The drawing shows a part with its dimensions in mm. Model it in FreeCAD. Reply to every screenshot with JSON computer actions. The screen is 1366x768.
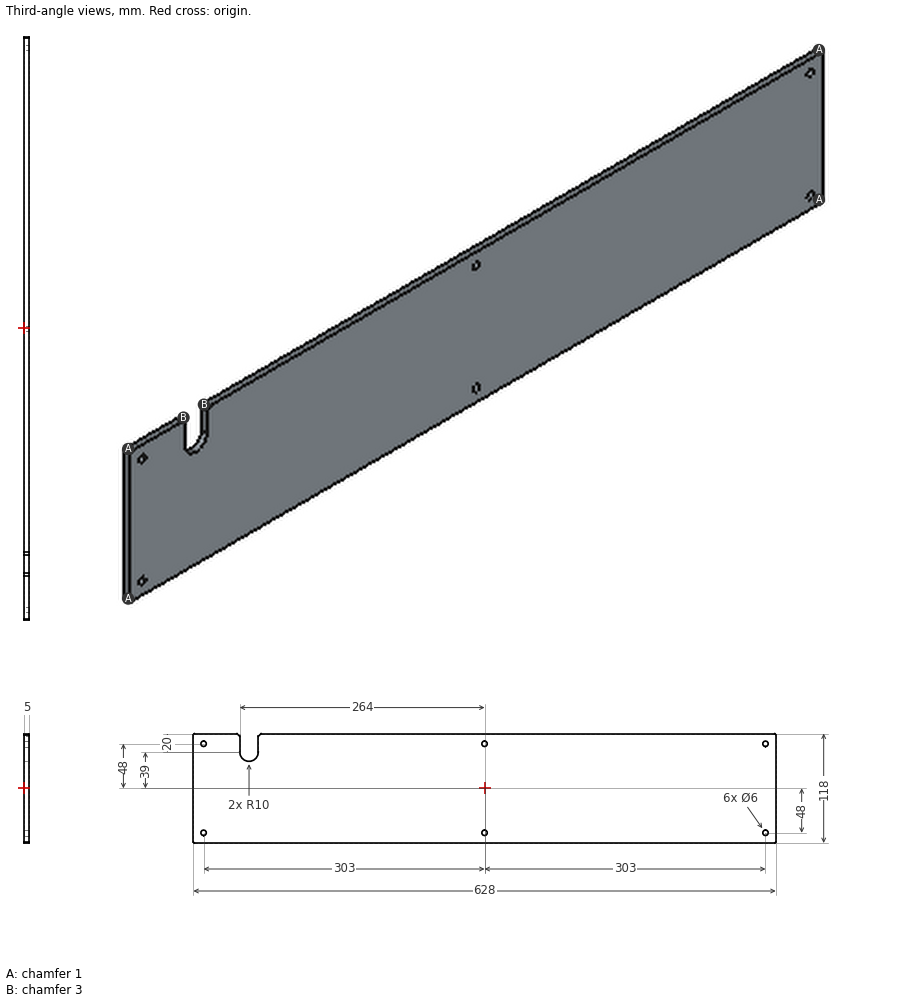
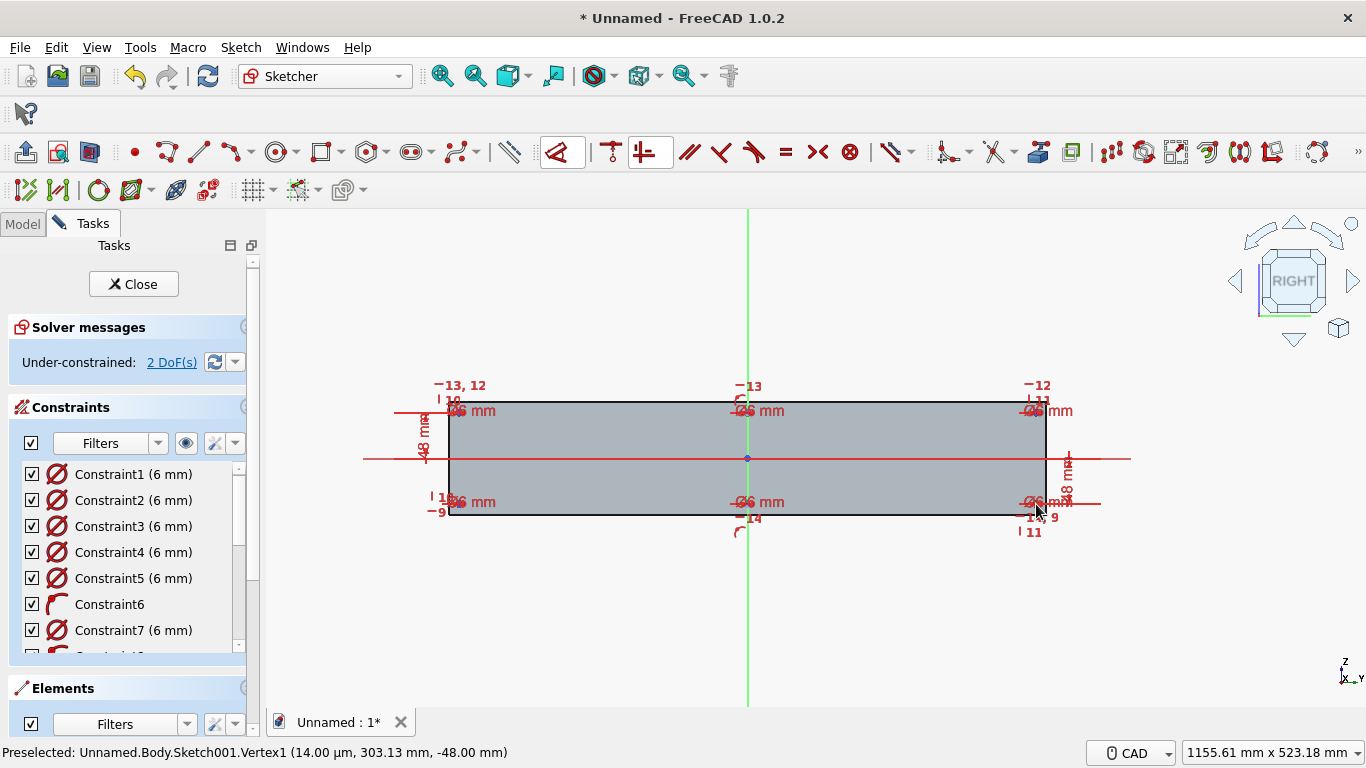
{"action": "left_click", "coordinate": [580, 152]}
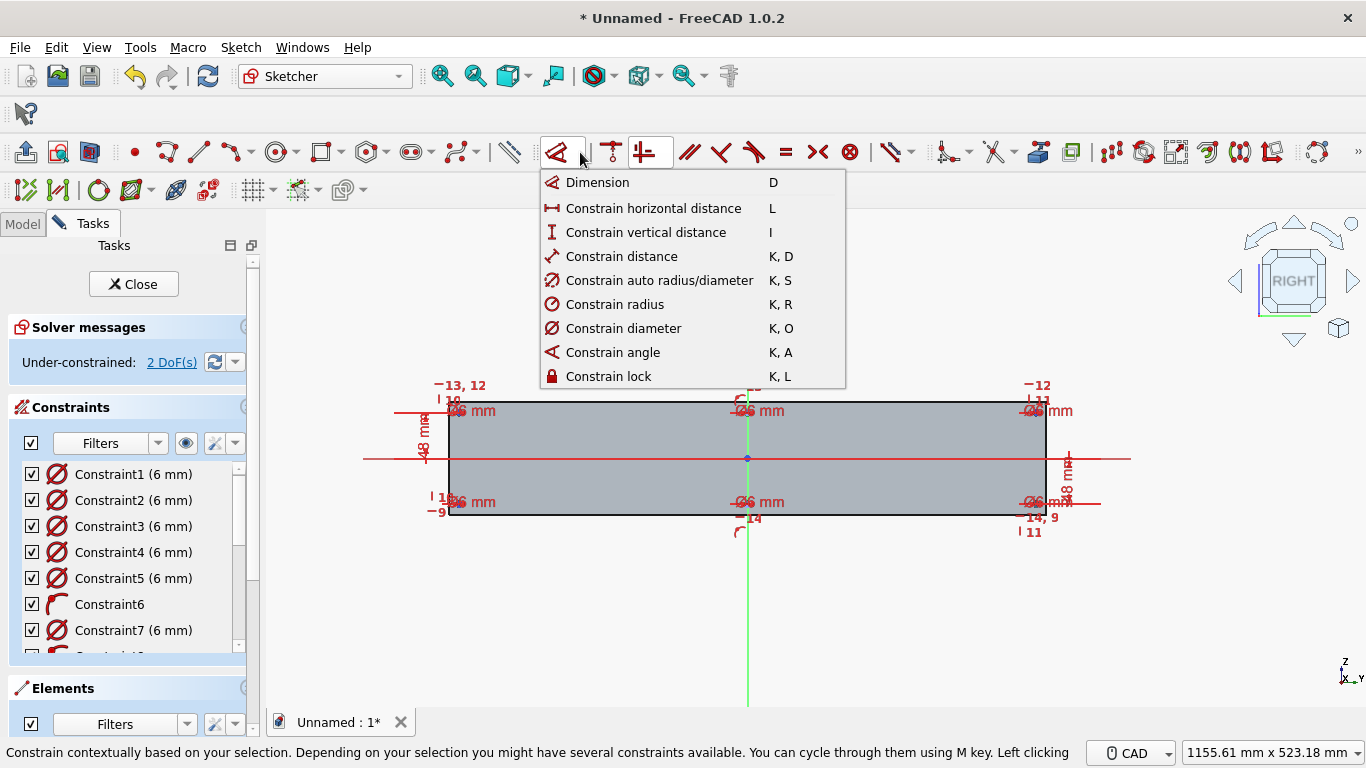
{"action": "left_click", "coordinate": [693, 208]}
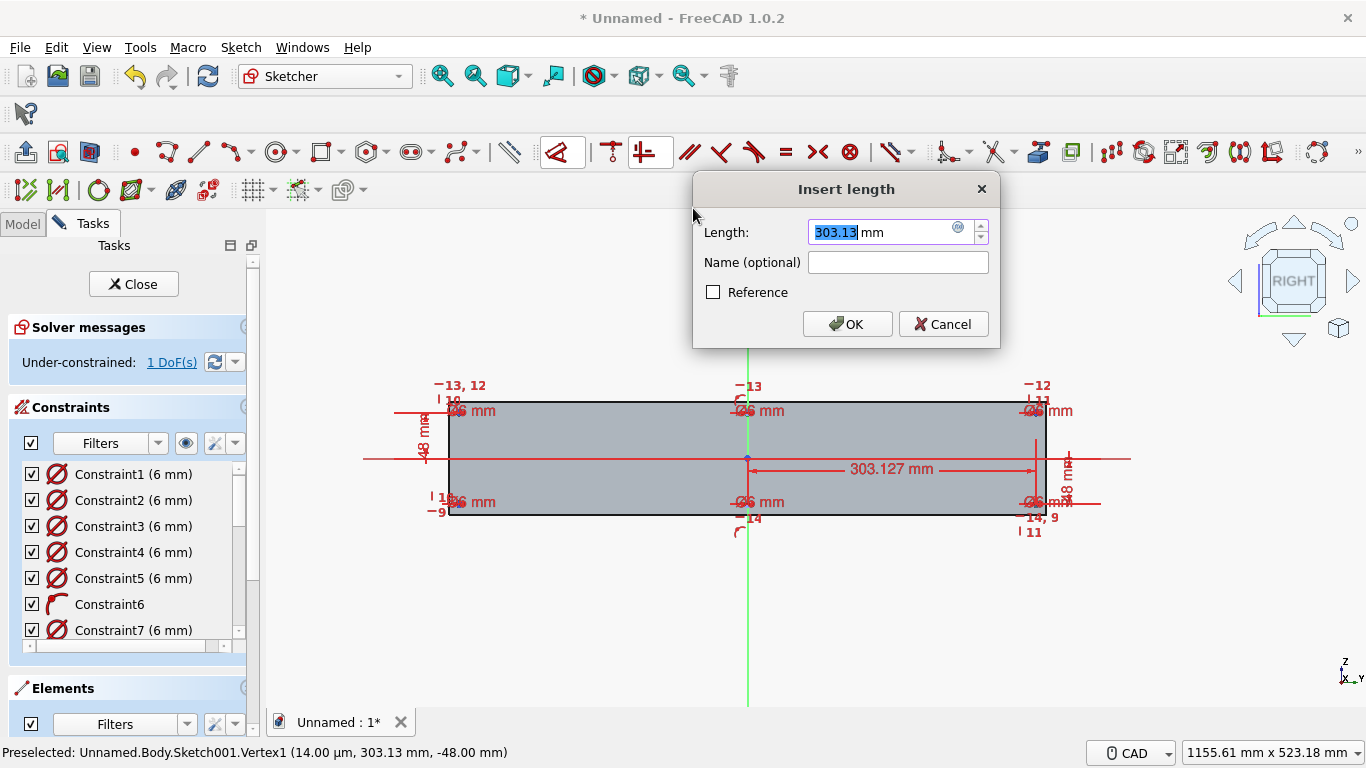
{"action": "type", "text": "303"}
{"action": "key", "text": "Return"}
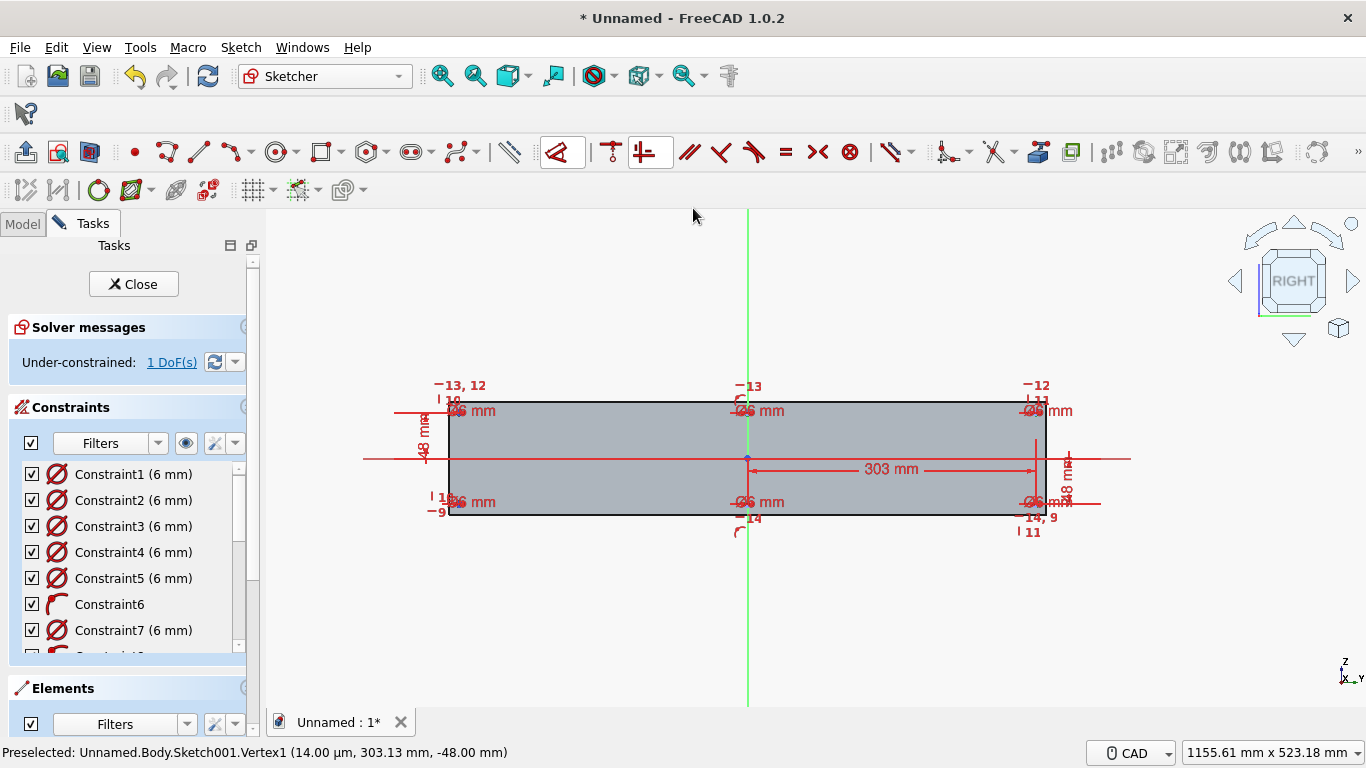
{"action": "left_click", "coordinate": [459, 504]}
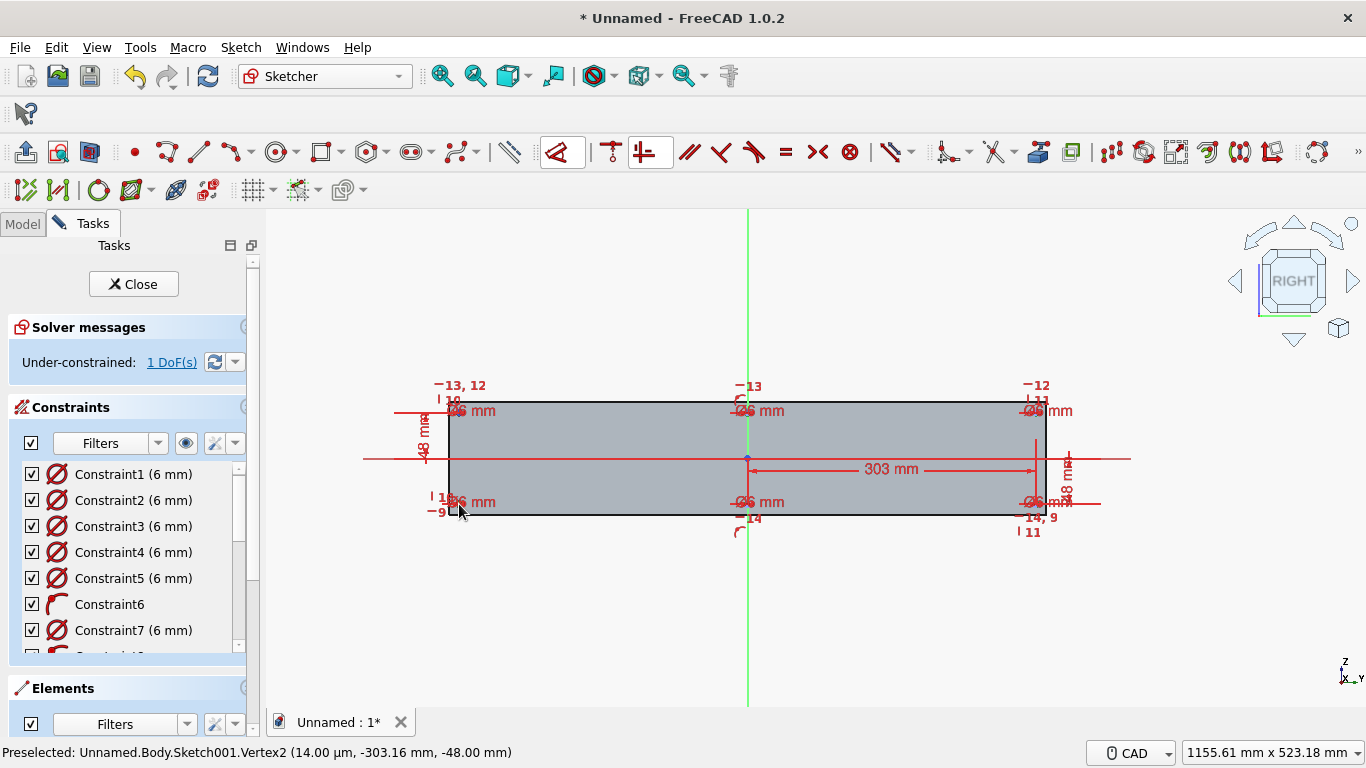
{"action": "left_click", "coordinate": [580, 152]}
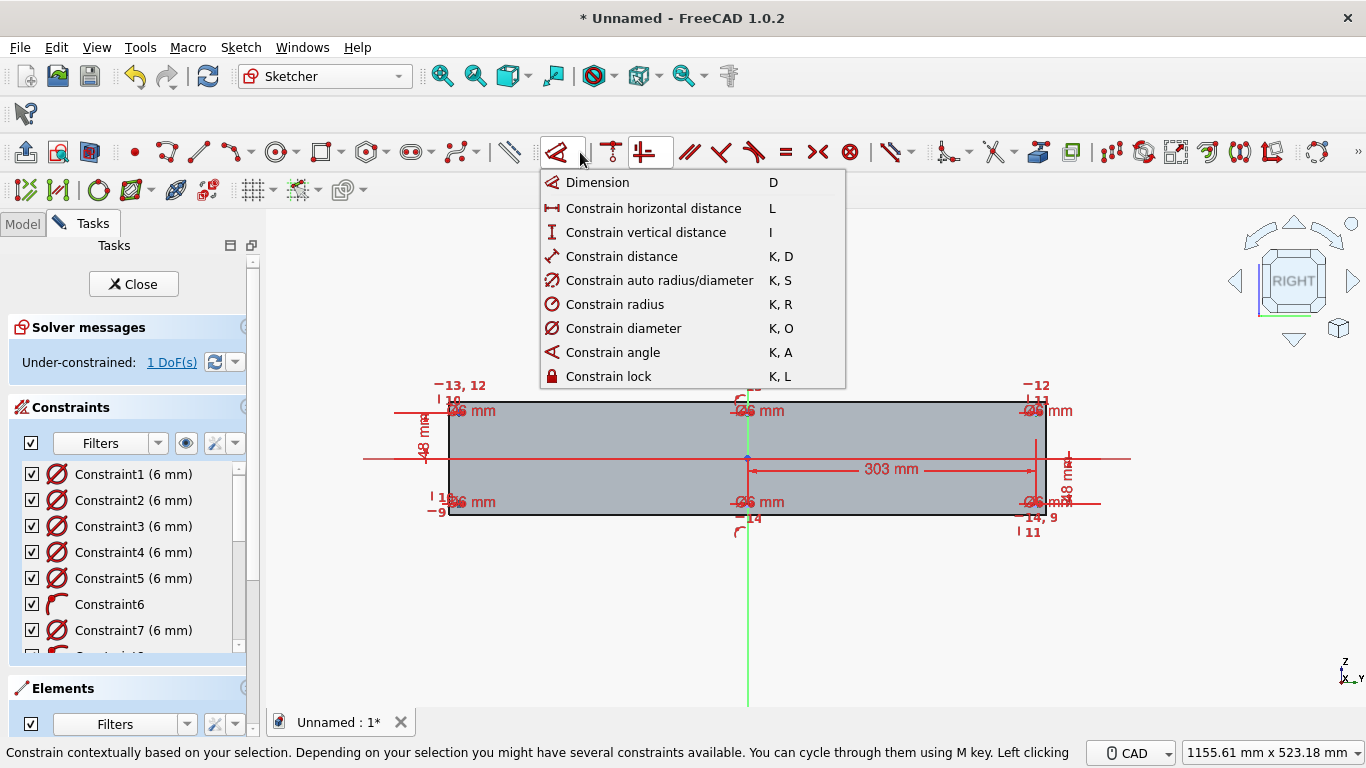
{"action": "left_click", "coordinate": [693, 208]}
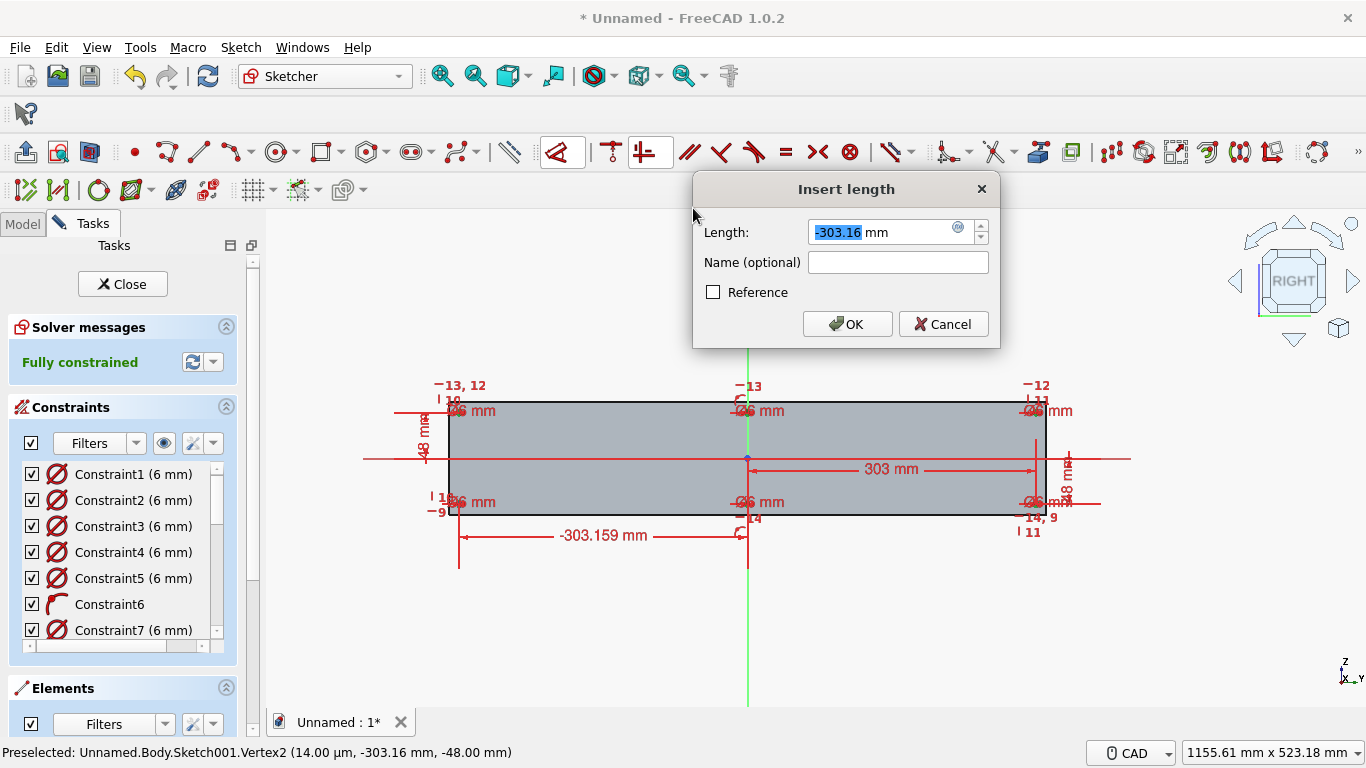
{"action": "type", "text": "-303"}
{"action": "key", "text": "Return"}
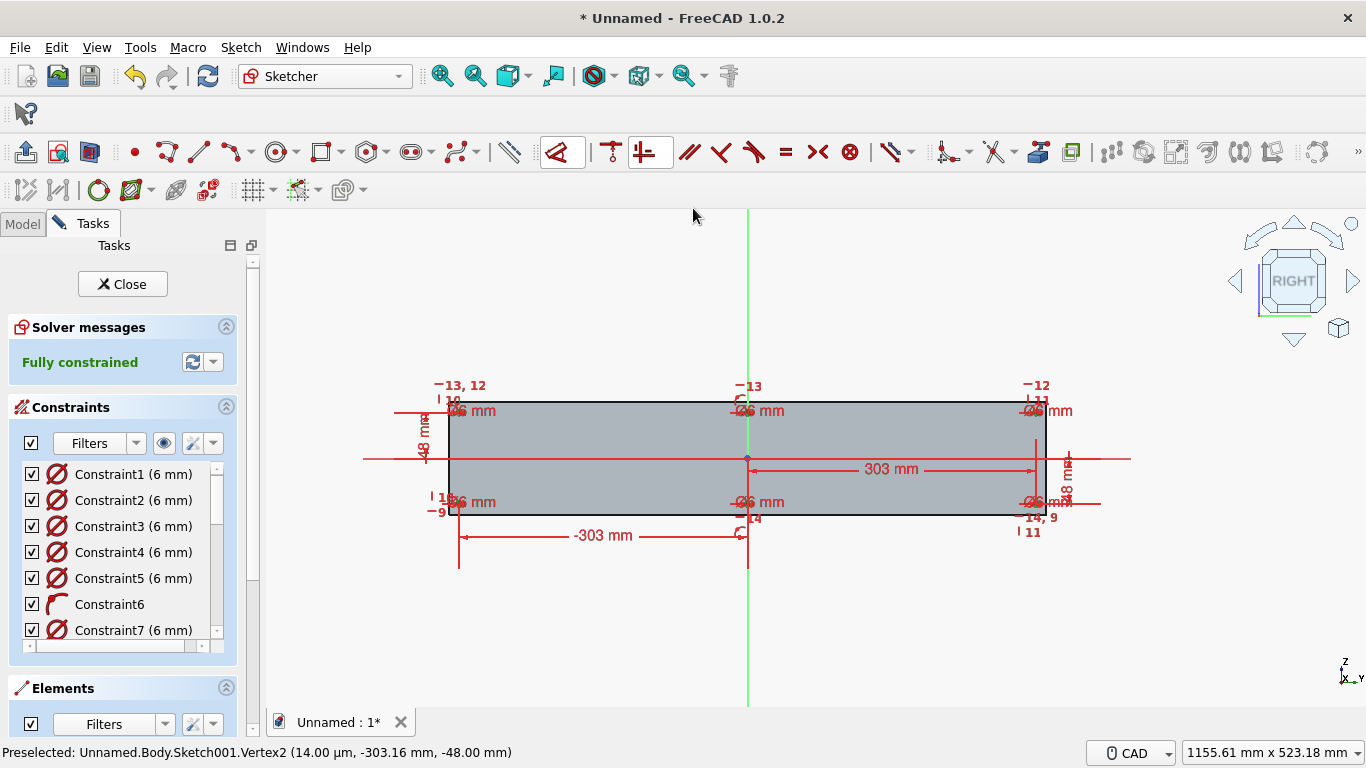
{"action": "left_click", "coordinate": [123, 284]}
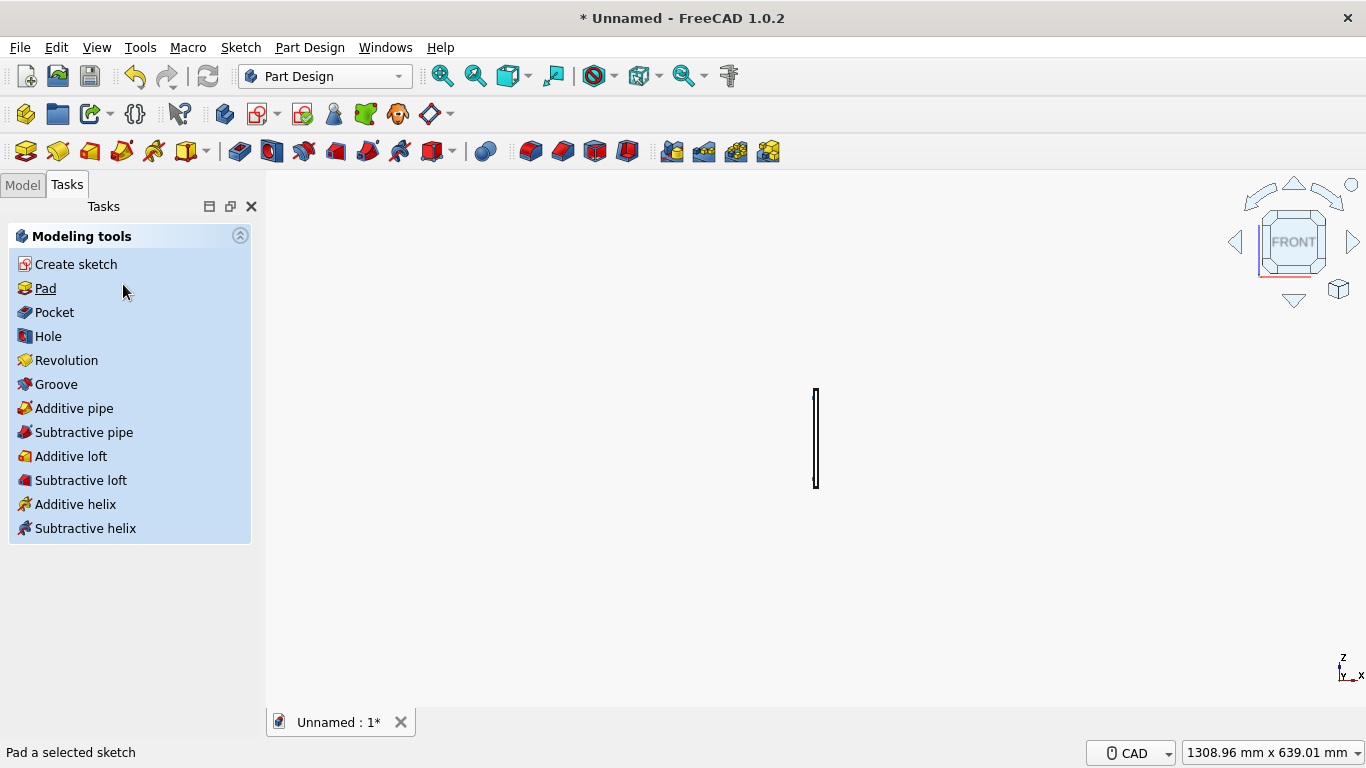
{"action": "left_click", "coordinate": [240, 152]}